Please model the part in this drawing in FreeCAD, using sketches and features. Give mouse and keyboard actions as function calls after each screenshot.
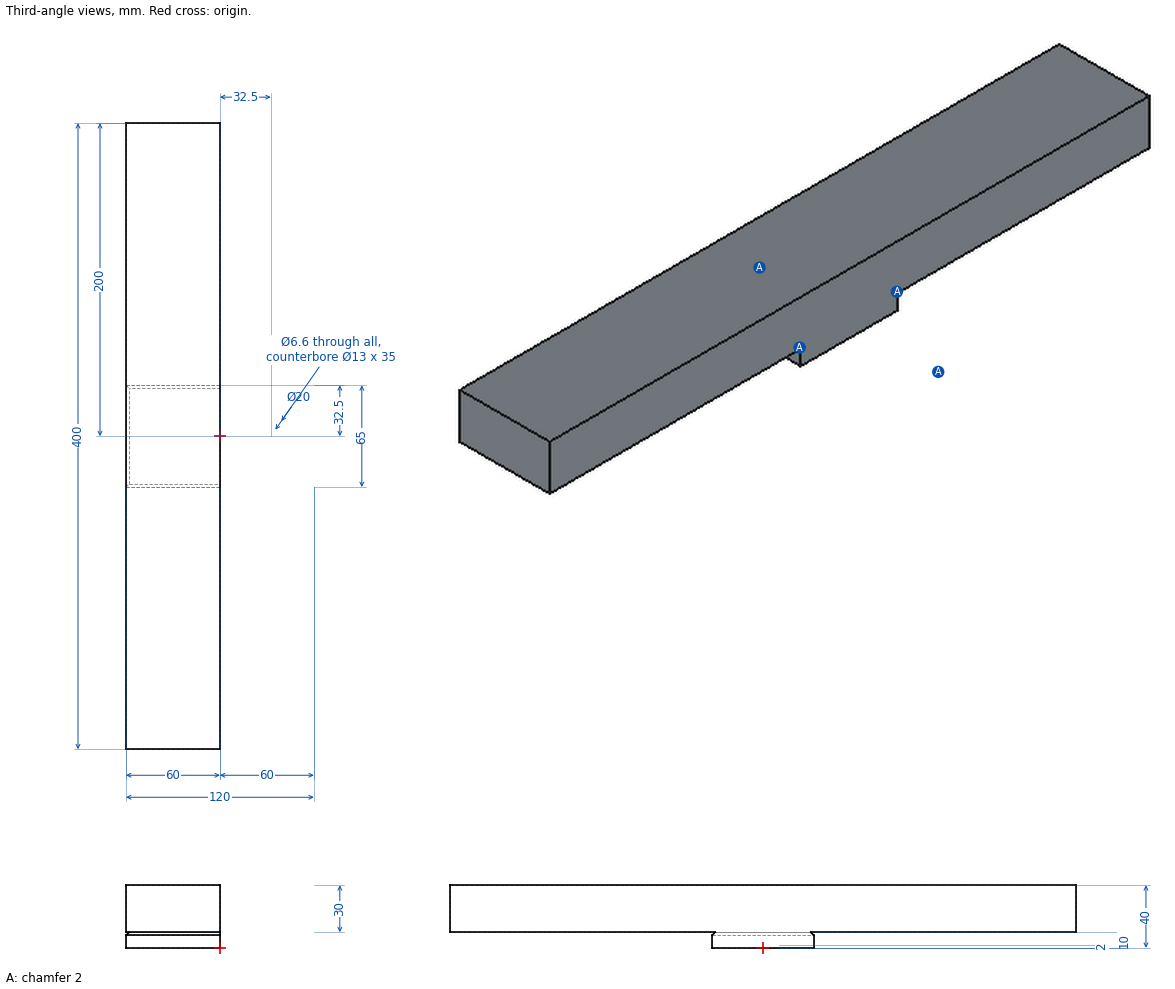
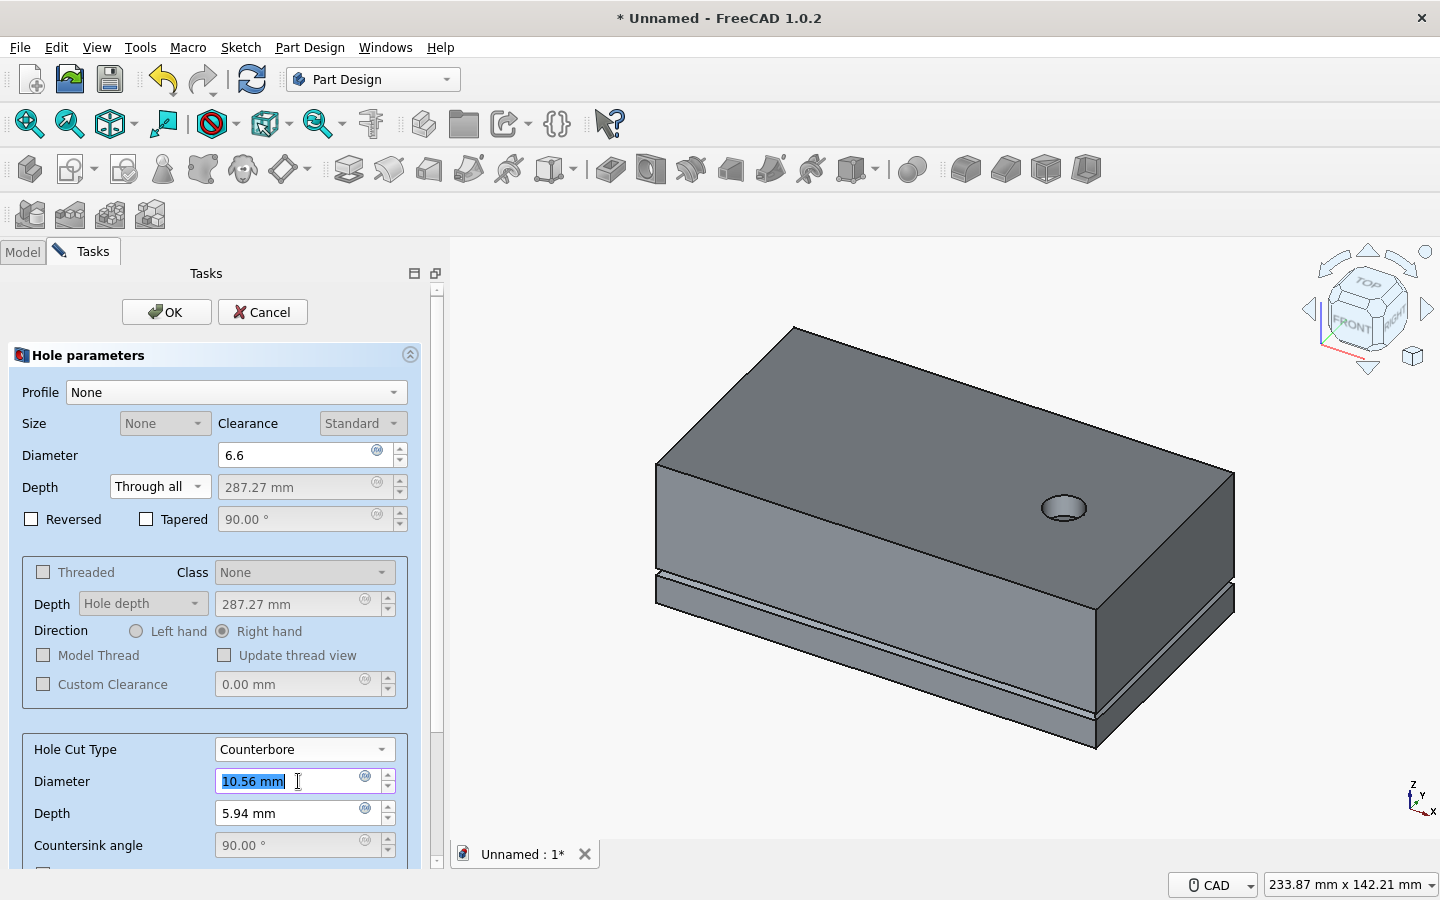
text(13)
key(Tab)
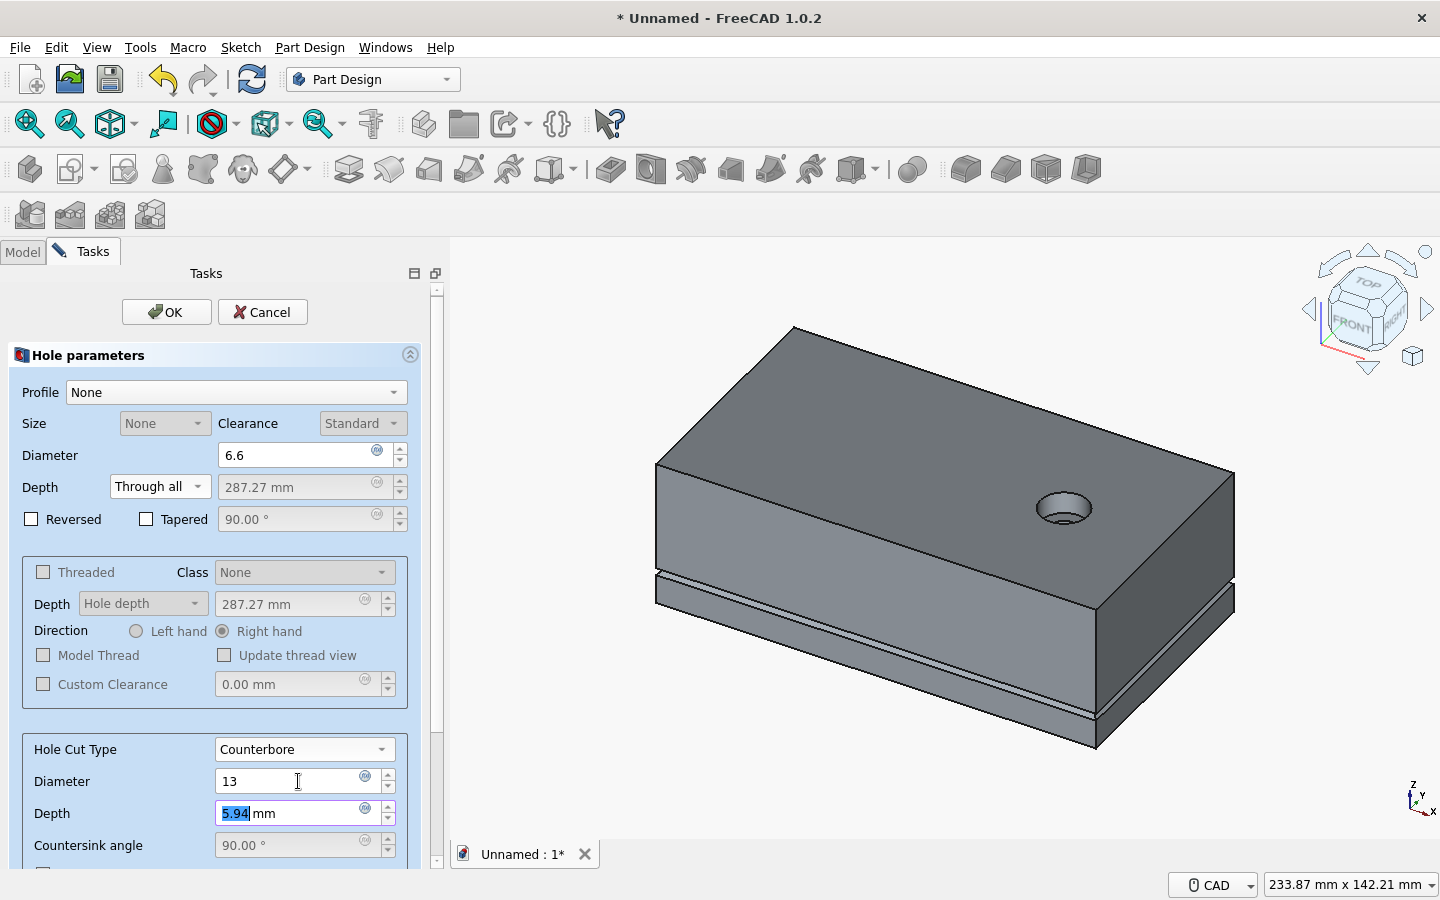
text(35)
key(Tab)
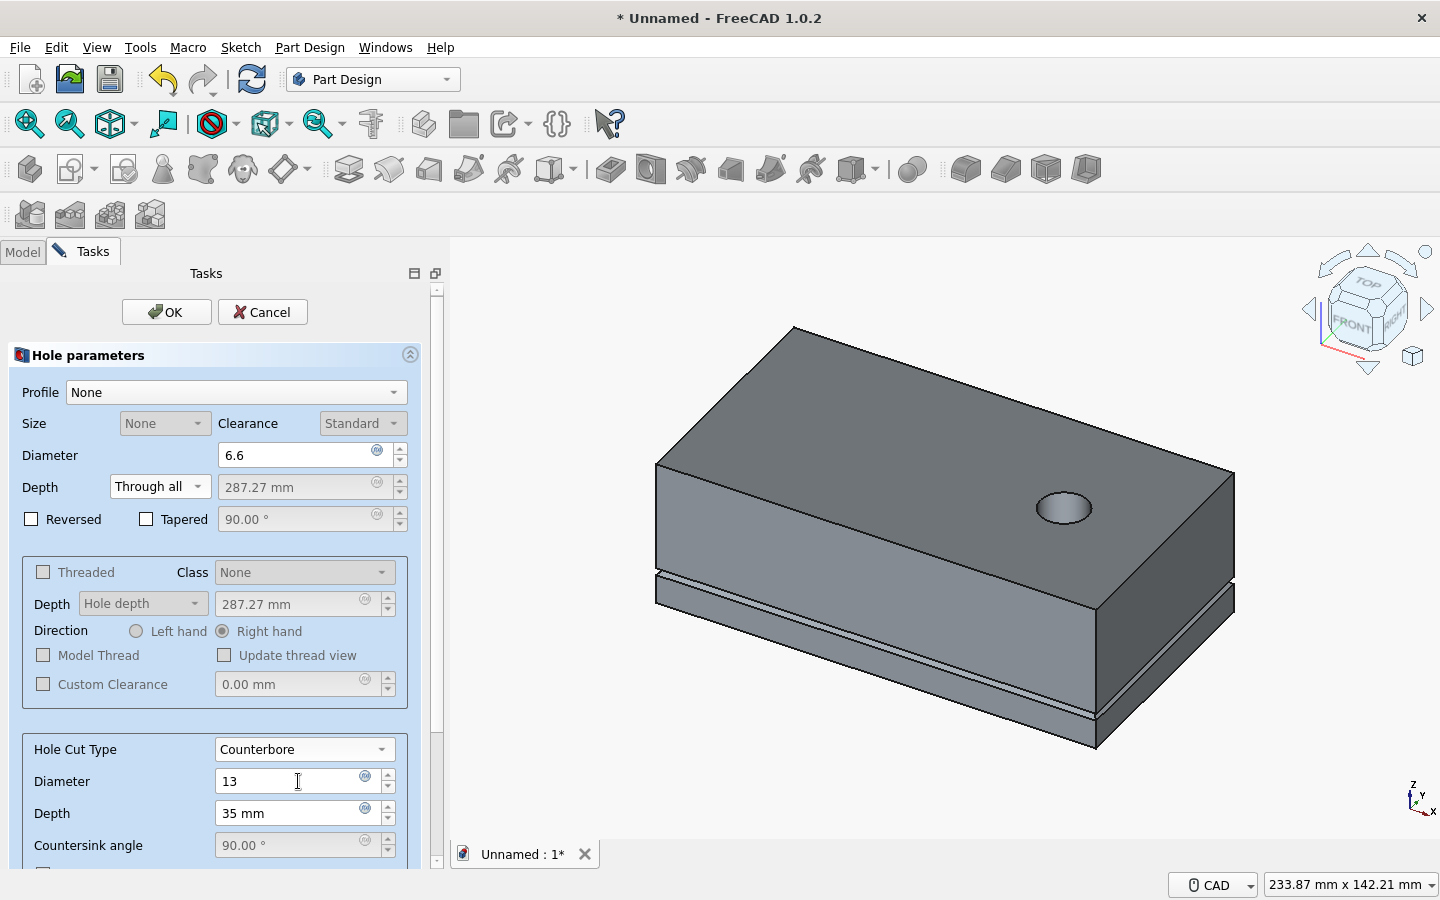
click(167, 312)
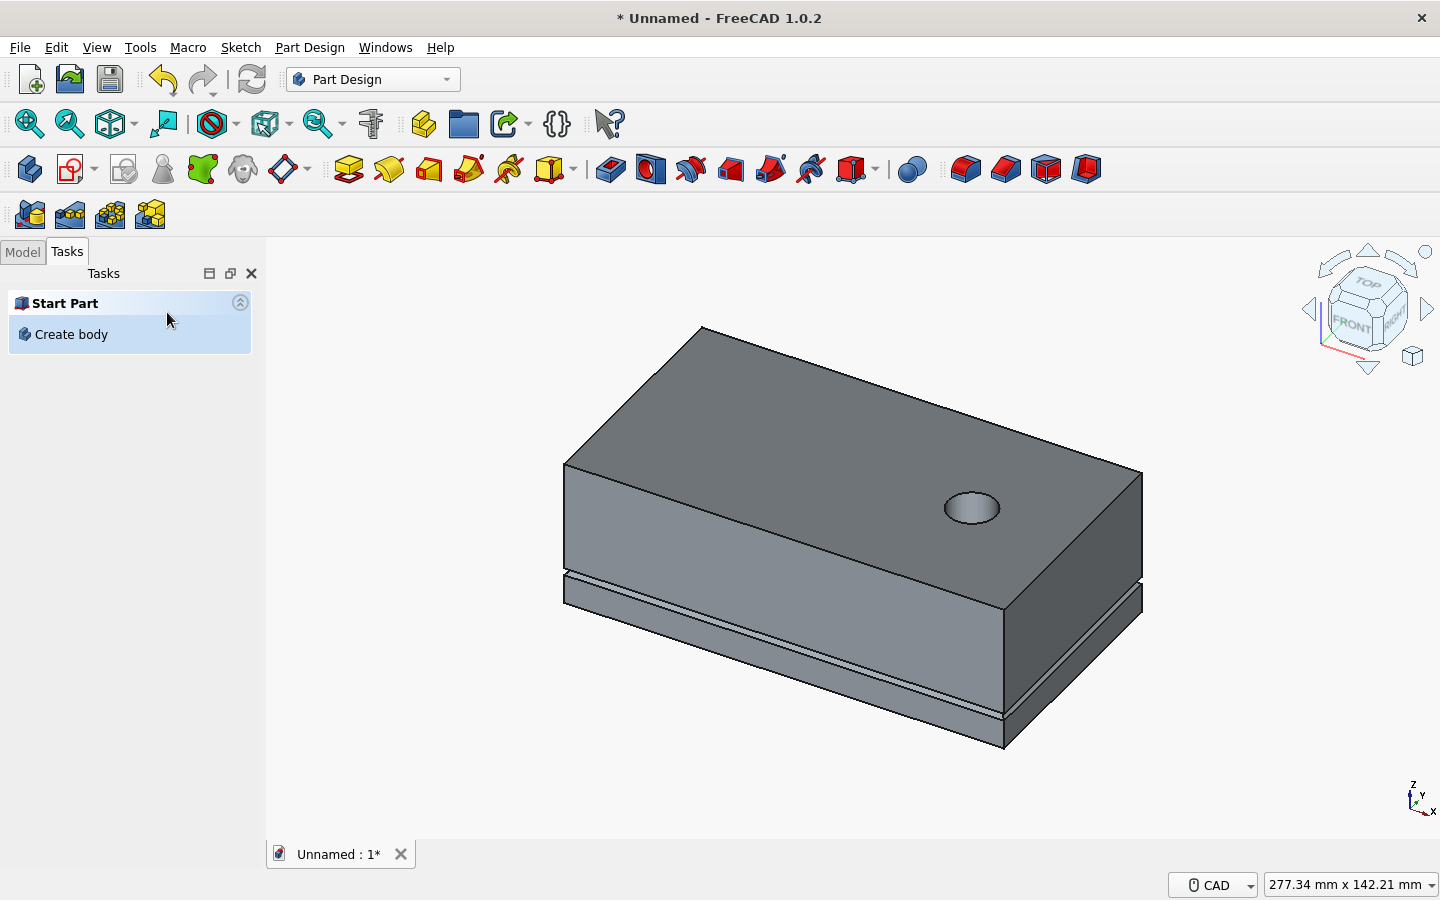
click(790, 447)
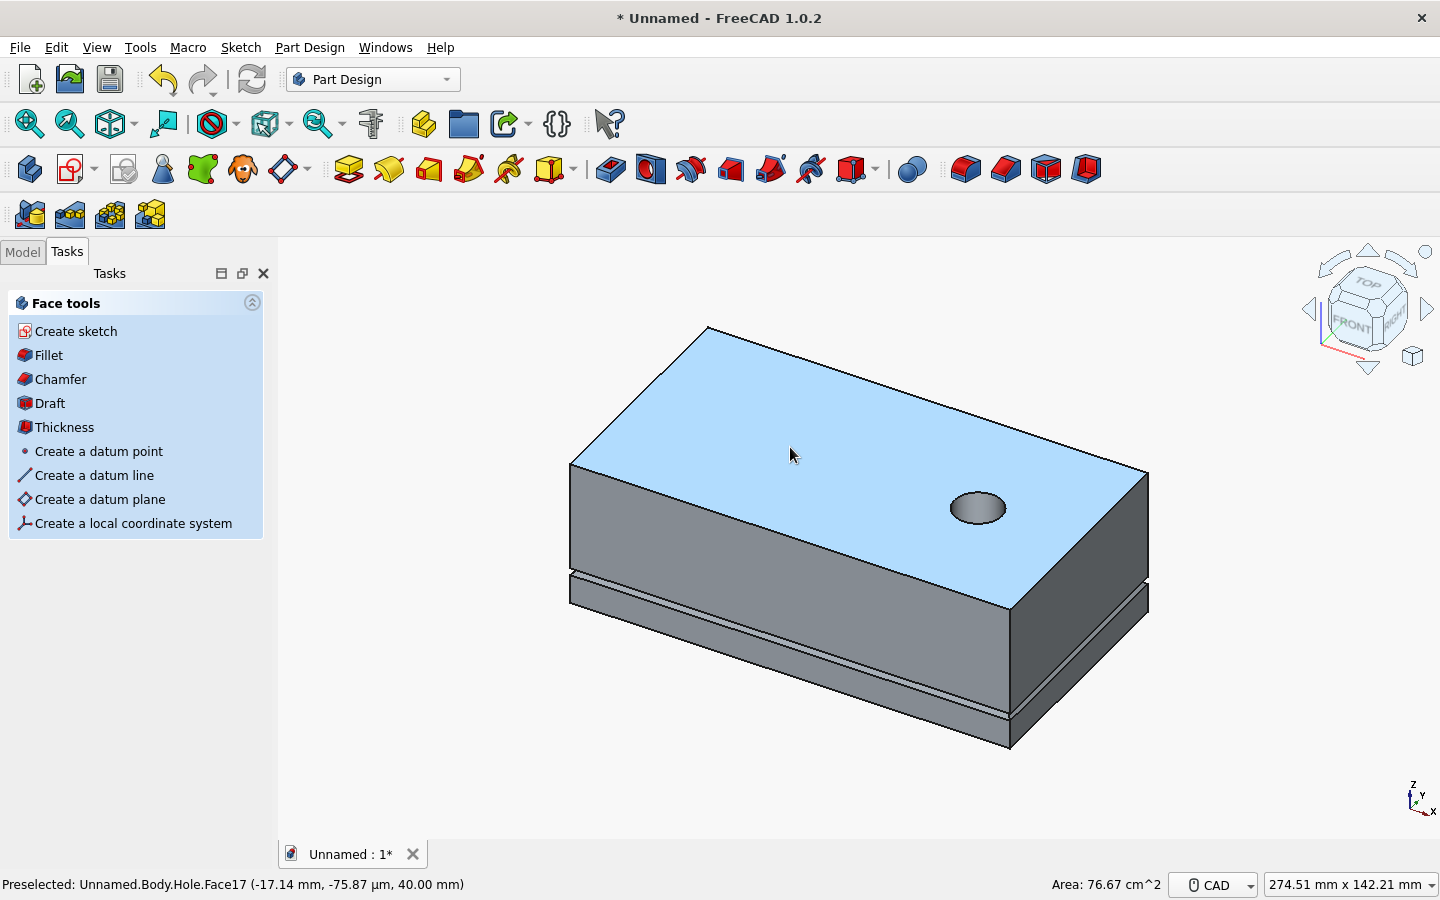
click(70, 170)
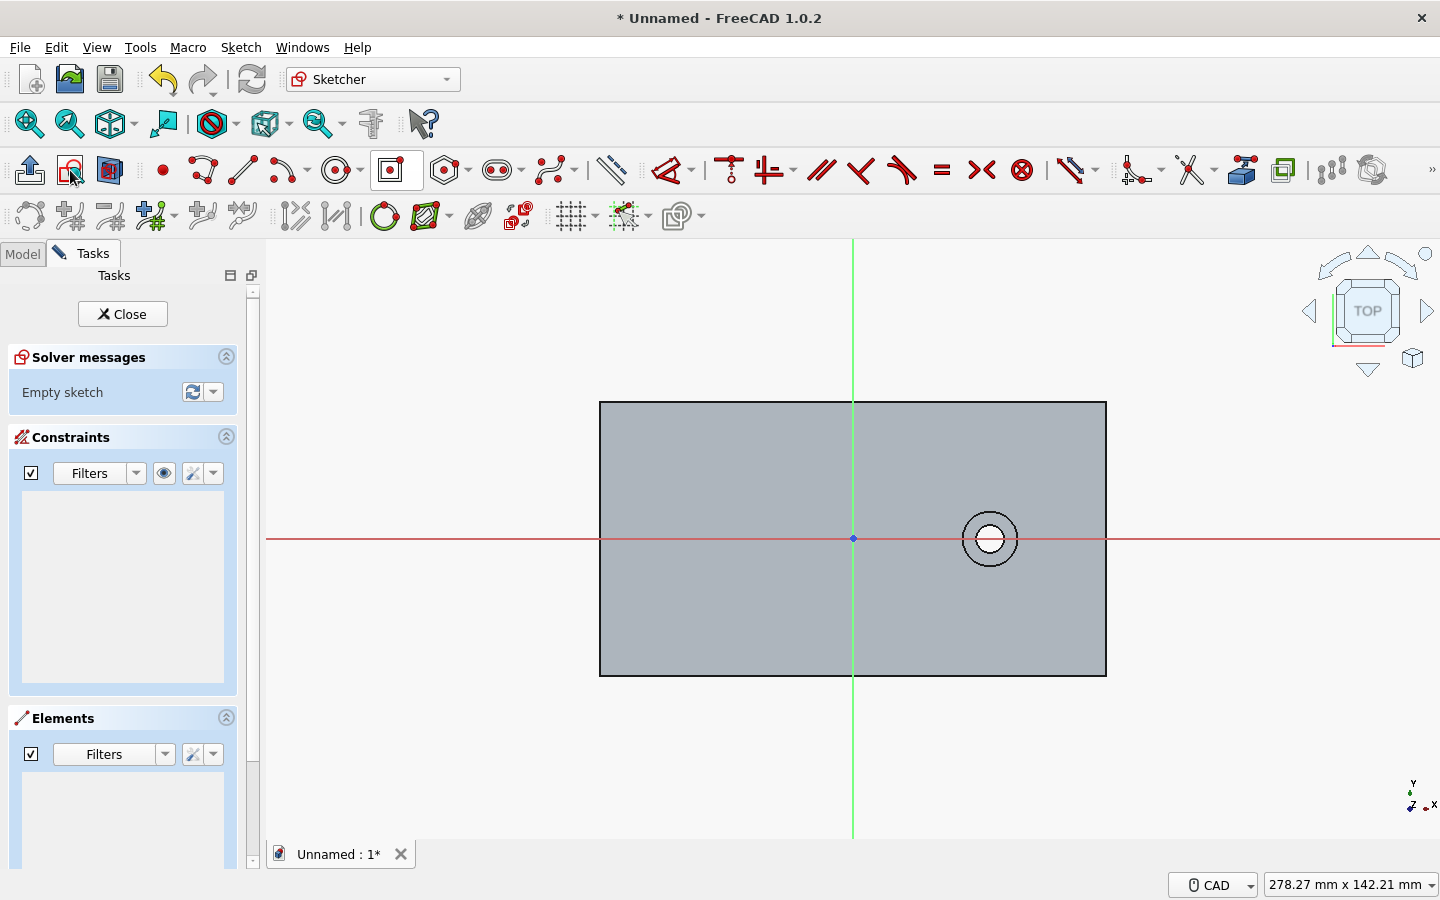
scroll(804, 539, down, 7)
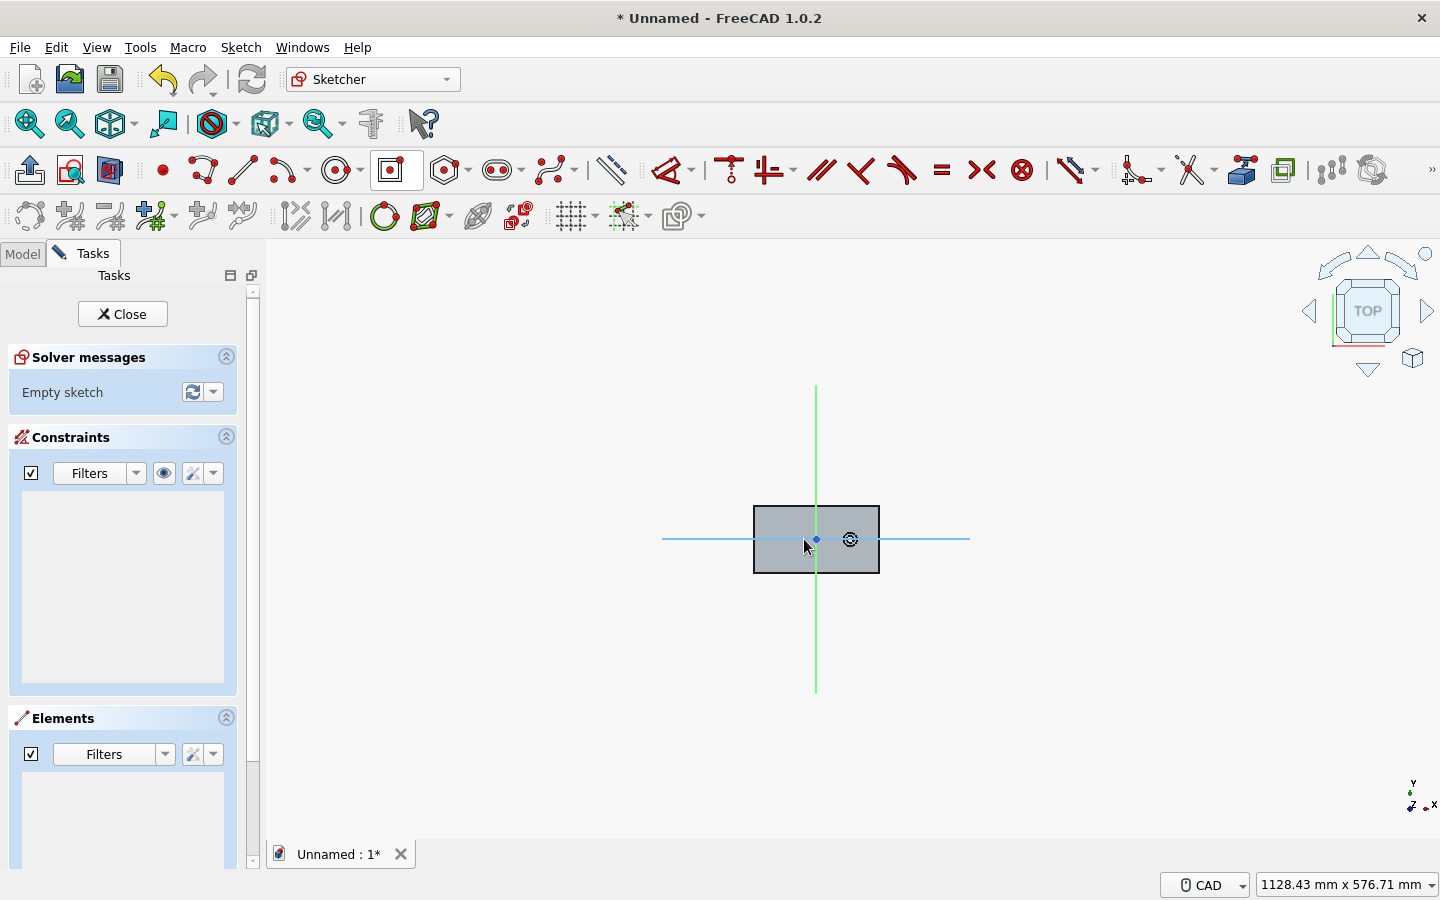
key(g)
key(r)